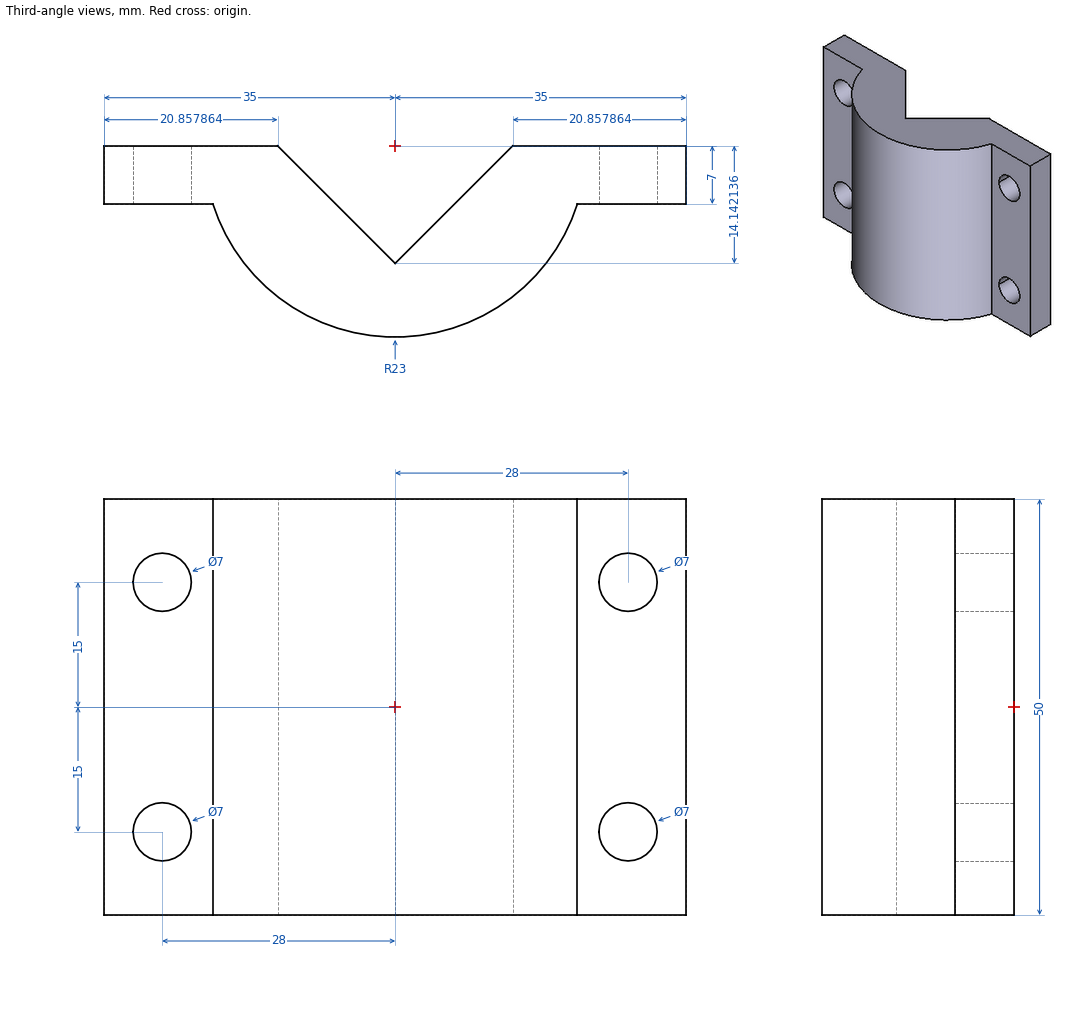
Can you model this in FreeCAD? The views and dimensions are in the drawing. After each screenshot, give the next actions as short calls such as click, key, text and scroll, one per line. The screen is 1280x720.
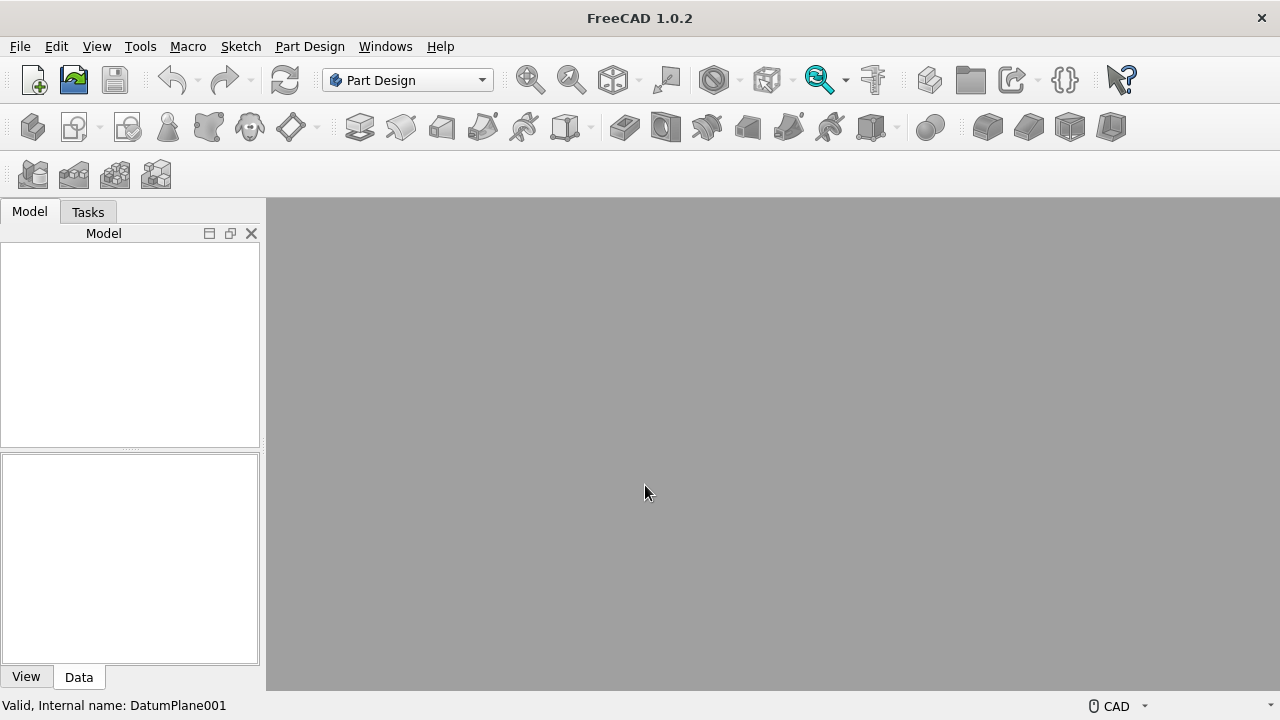
key(ctrl+n)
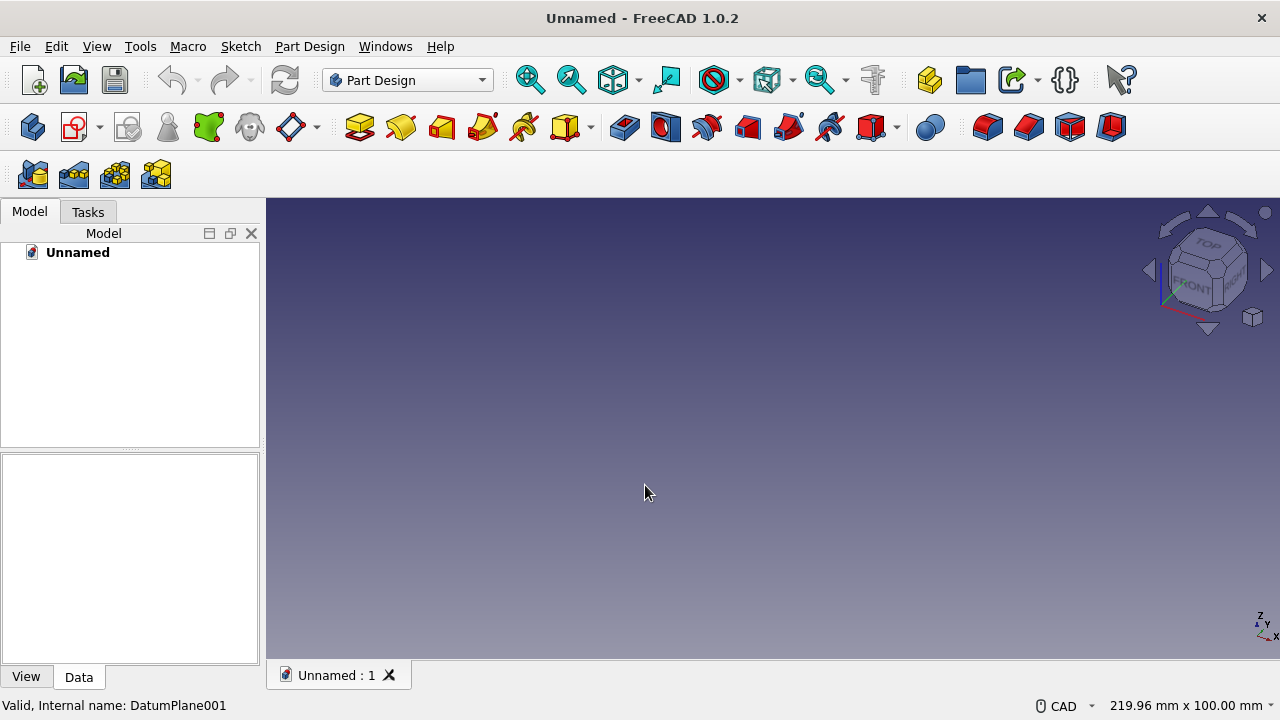
click(74, 128)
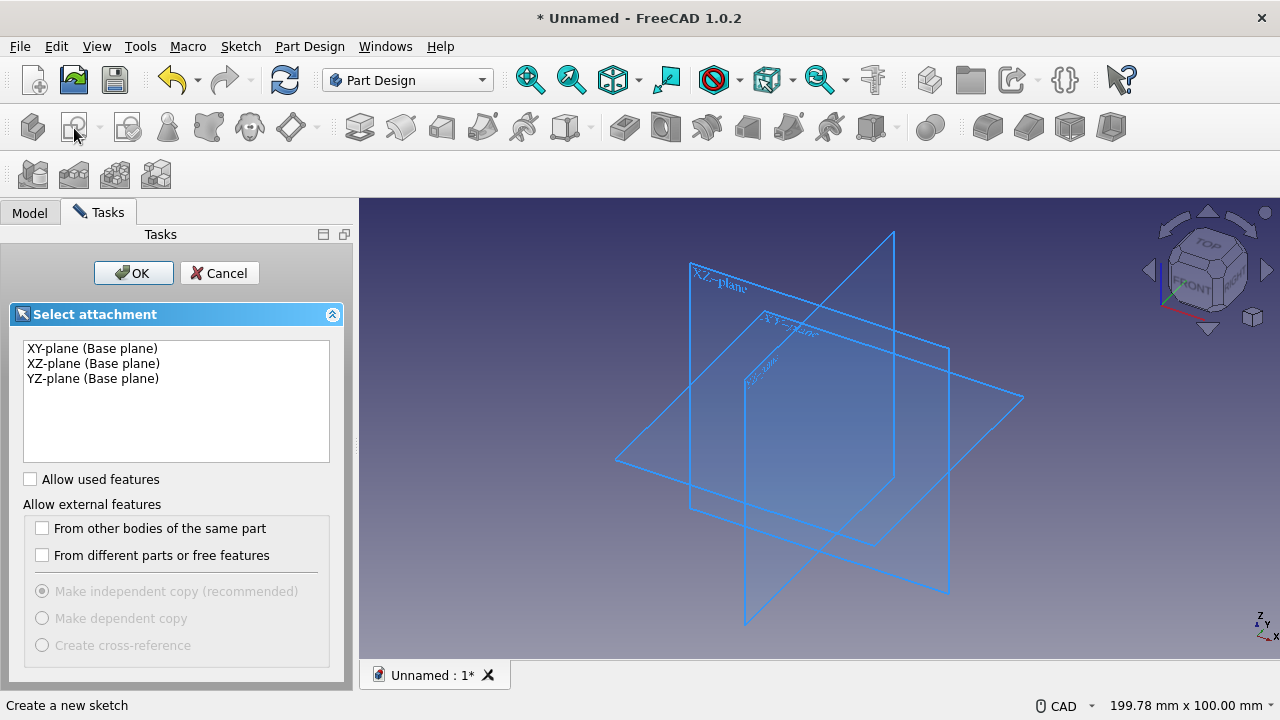
click(84, 348)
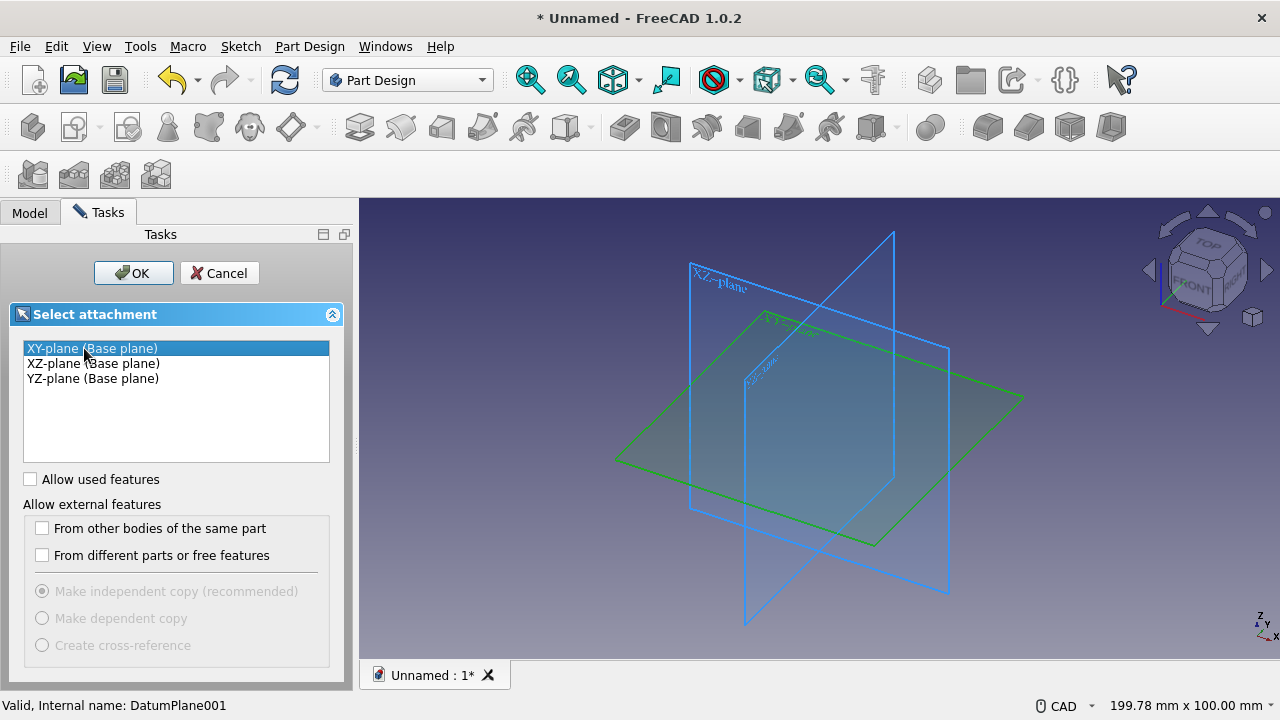
click(134, 273)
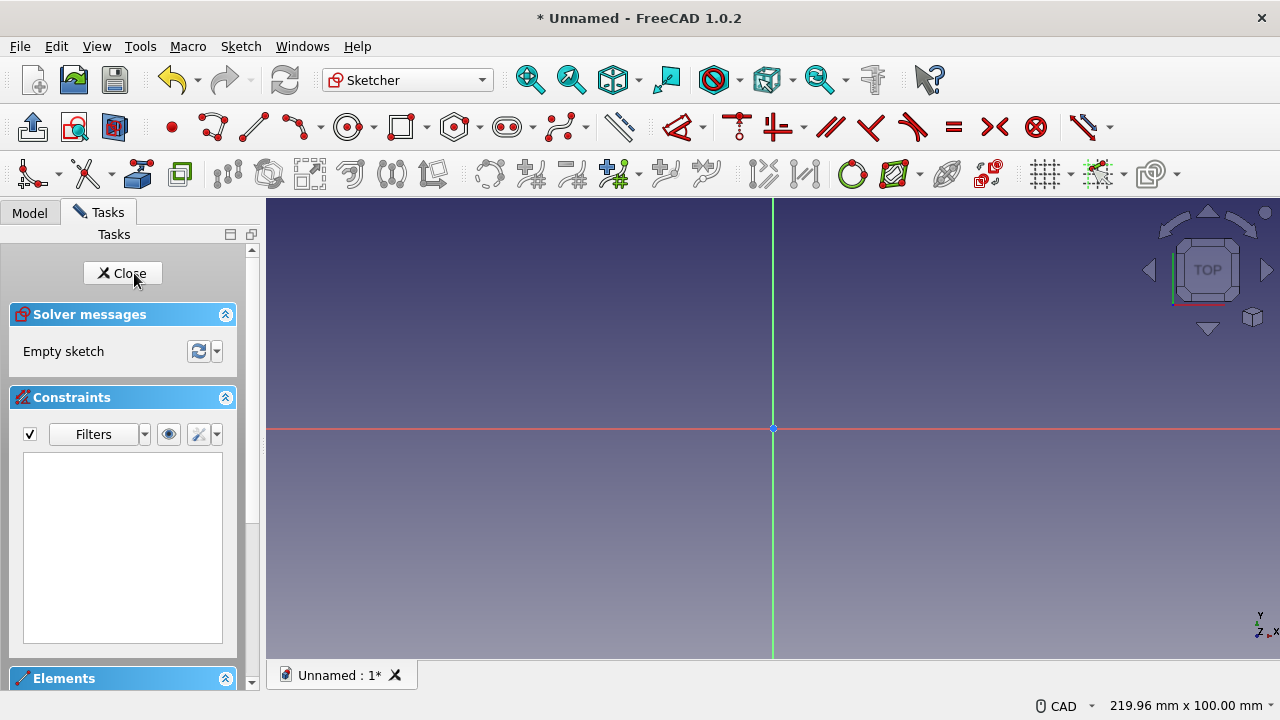
scroll(856, 546, up, 3)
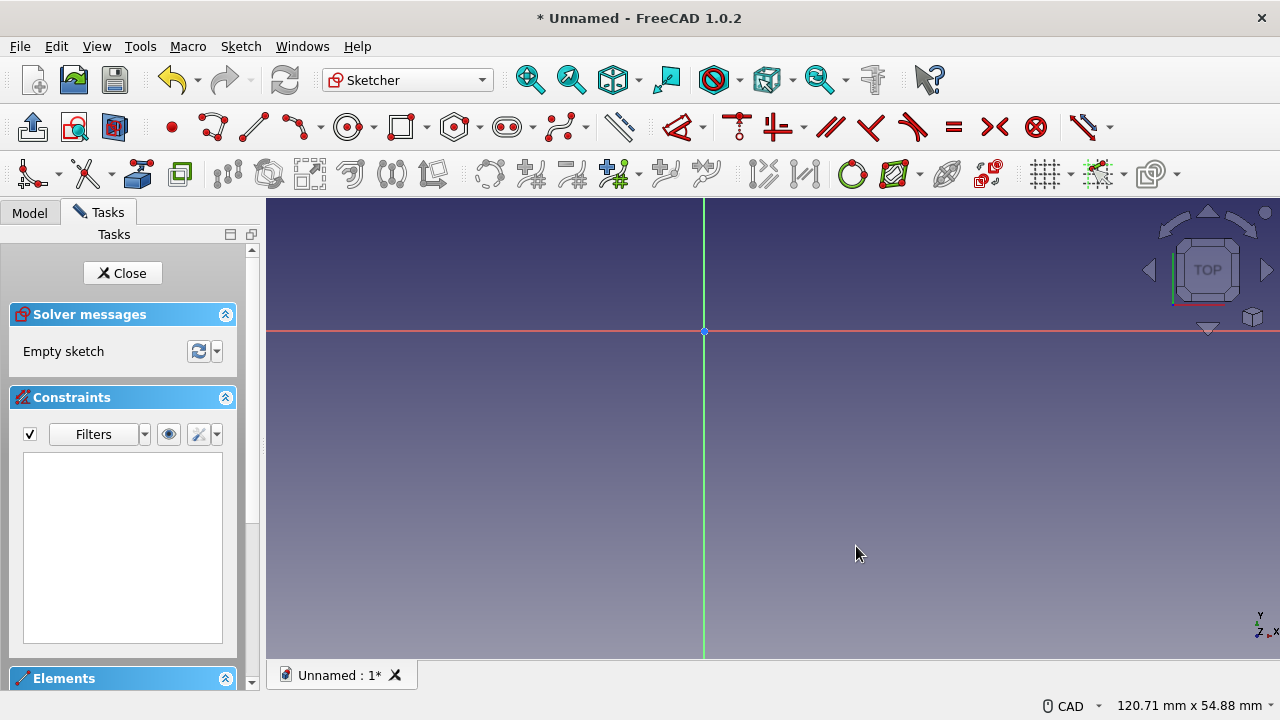
key(g)
key(m)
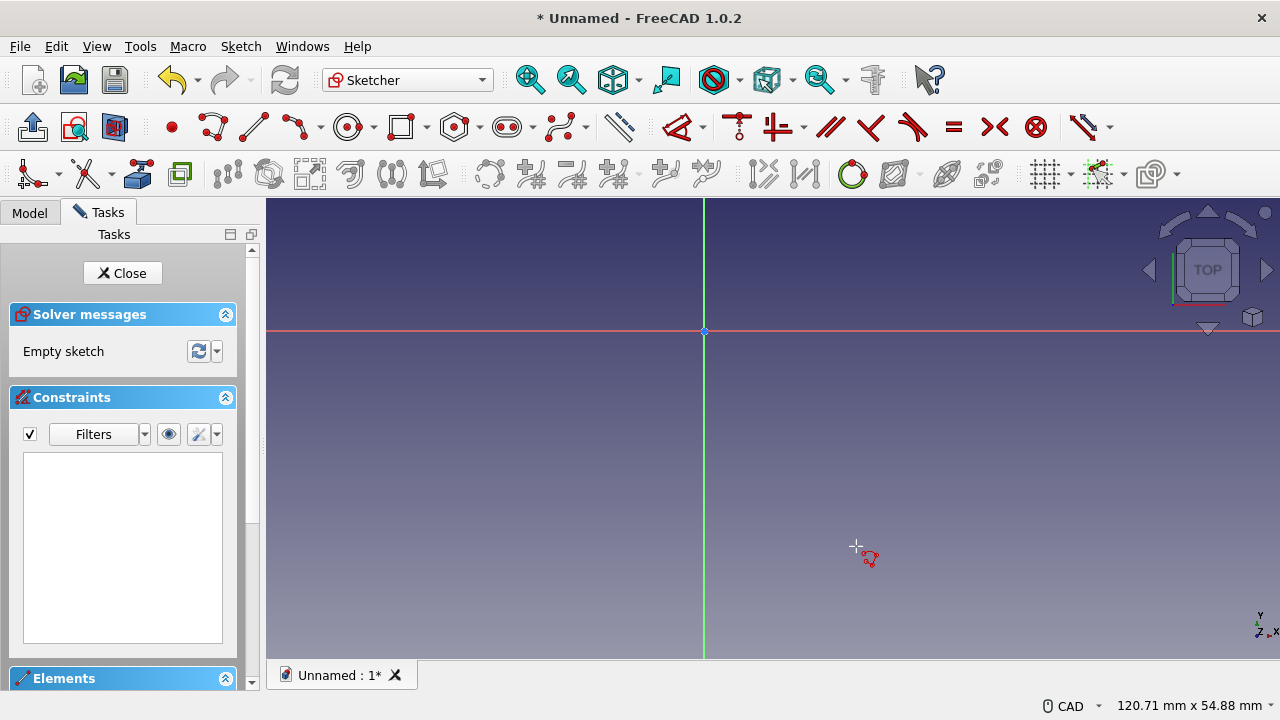
click(888, 390)
click(998, 390)
click(998, 331)
click(823, 340)
click(704, 450)
click(585, 331)
click(410, 340)
click(410, 390)
click(520, 390)
right_click(520, 390)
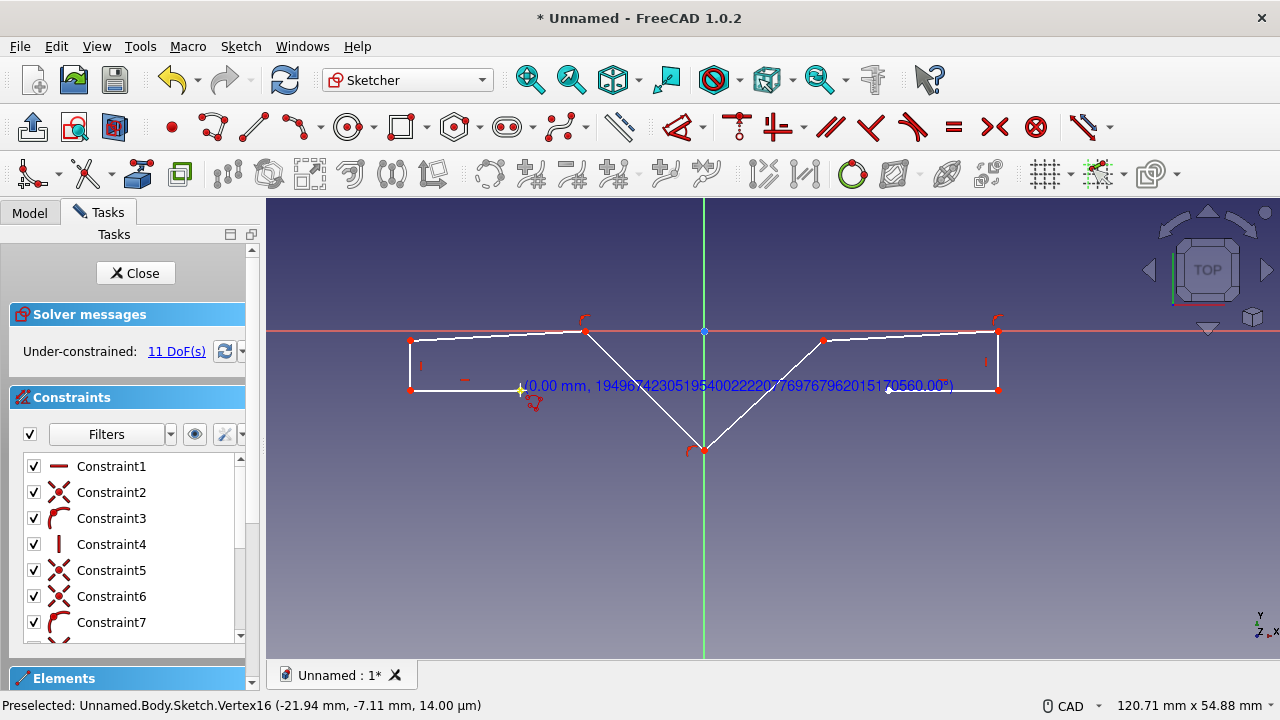
key(g)
key(3)
key(a)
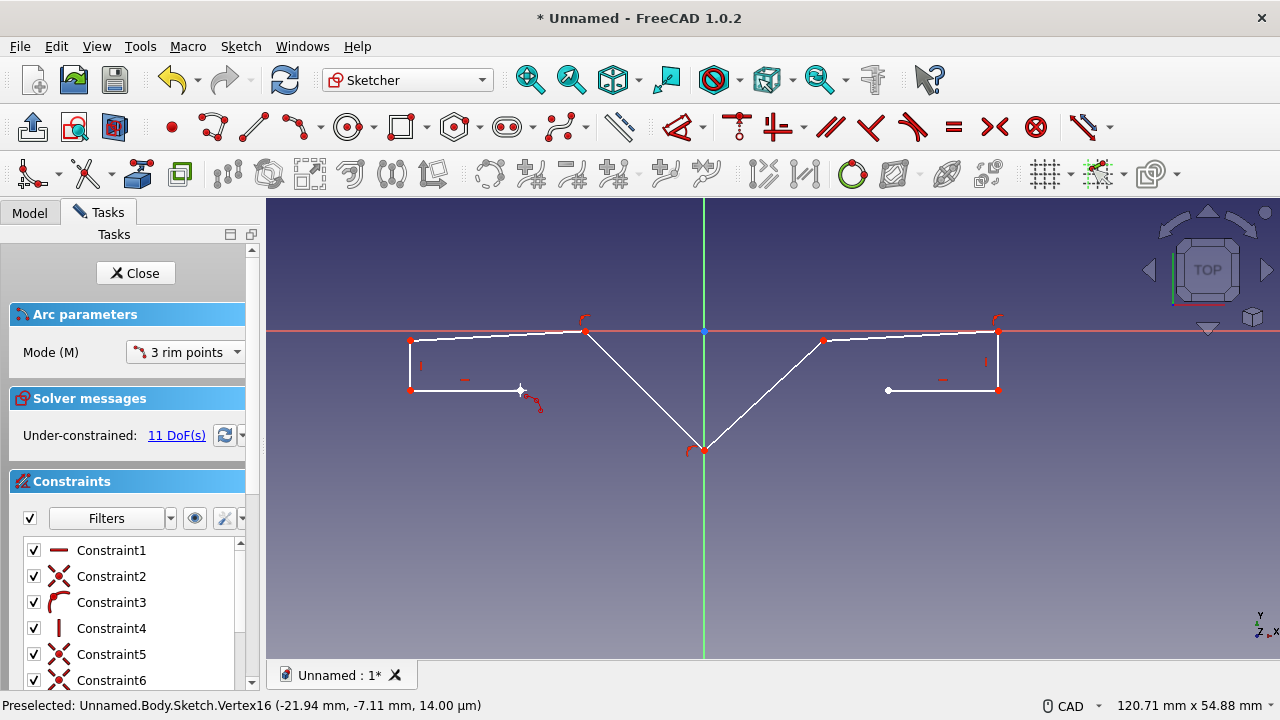
click(520, 391)
click(888, 391)
click(656, 518)
key(Escape)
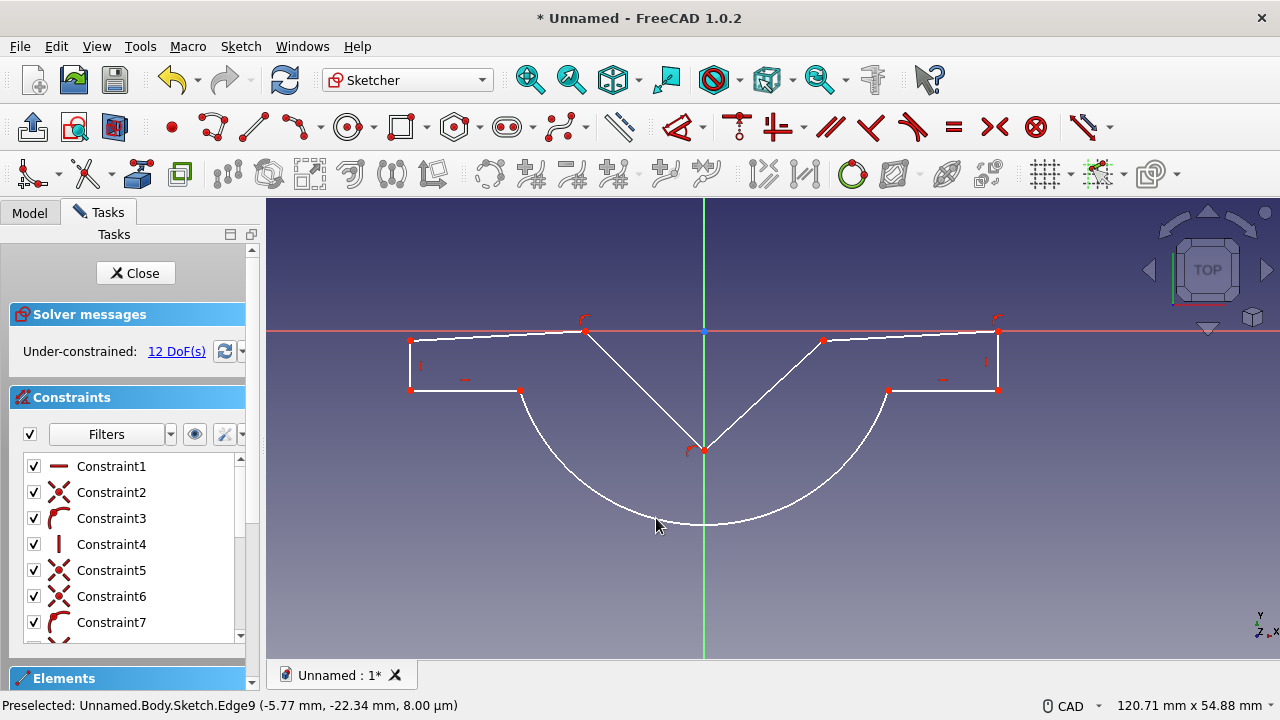
click(945, 334)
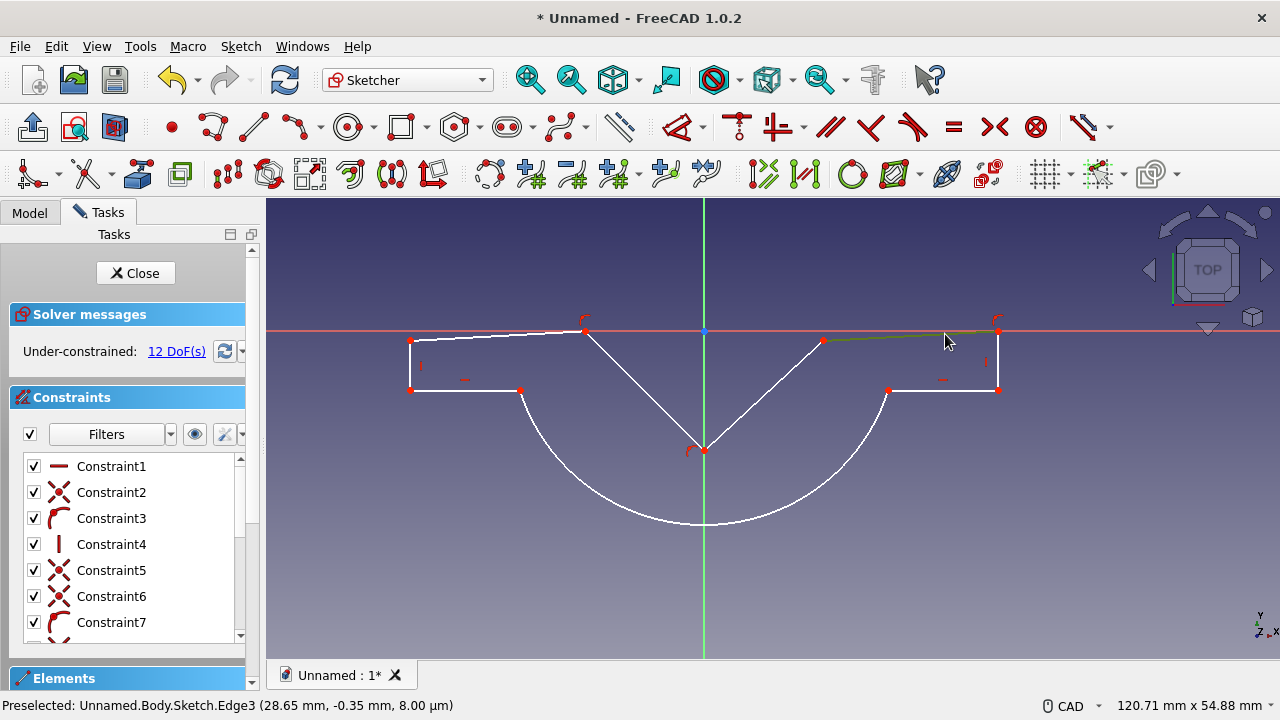
key(h)